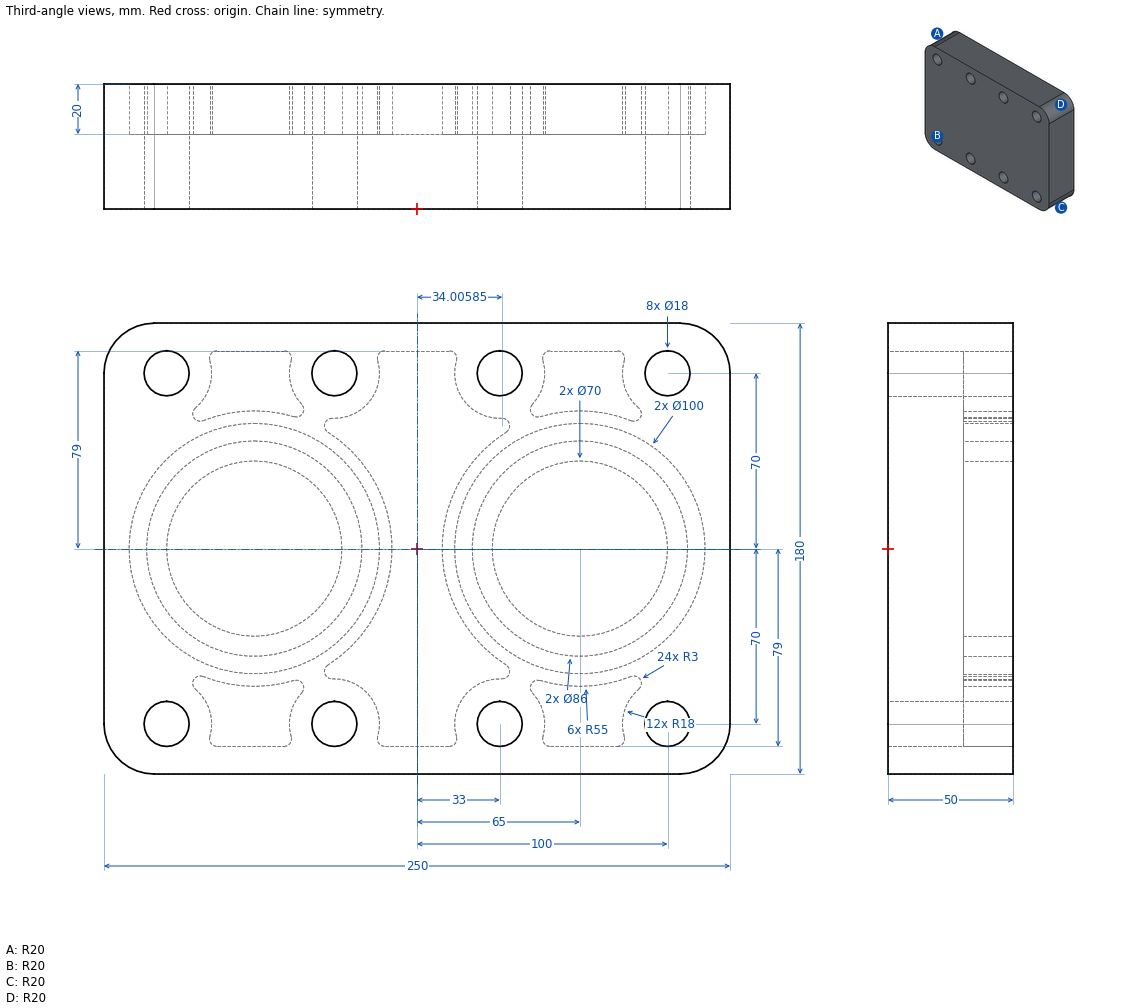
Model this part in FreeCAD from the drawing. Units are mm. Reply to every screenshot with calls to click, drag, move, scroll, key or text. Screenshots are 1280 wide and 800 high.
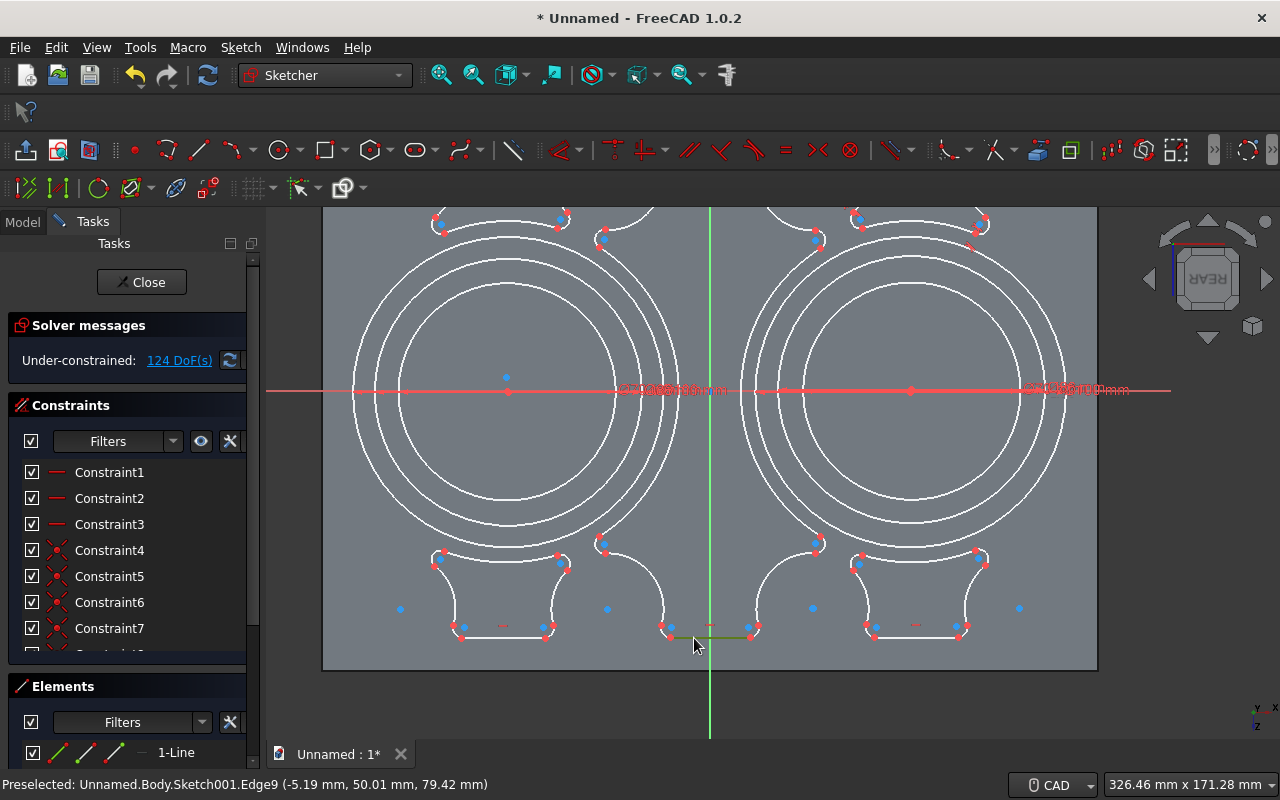
scroll(757, 633, up, 3)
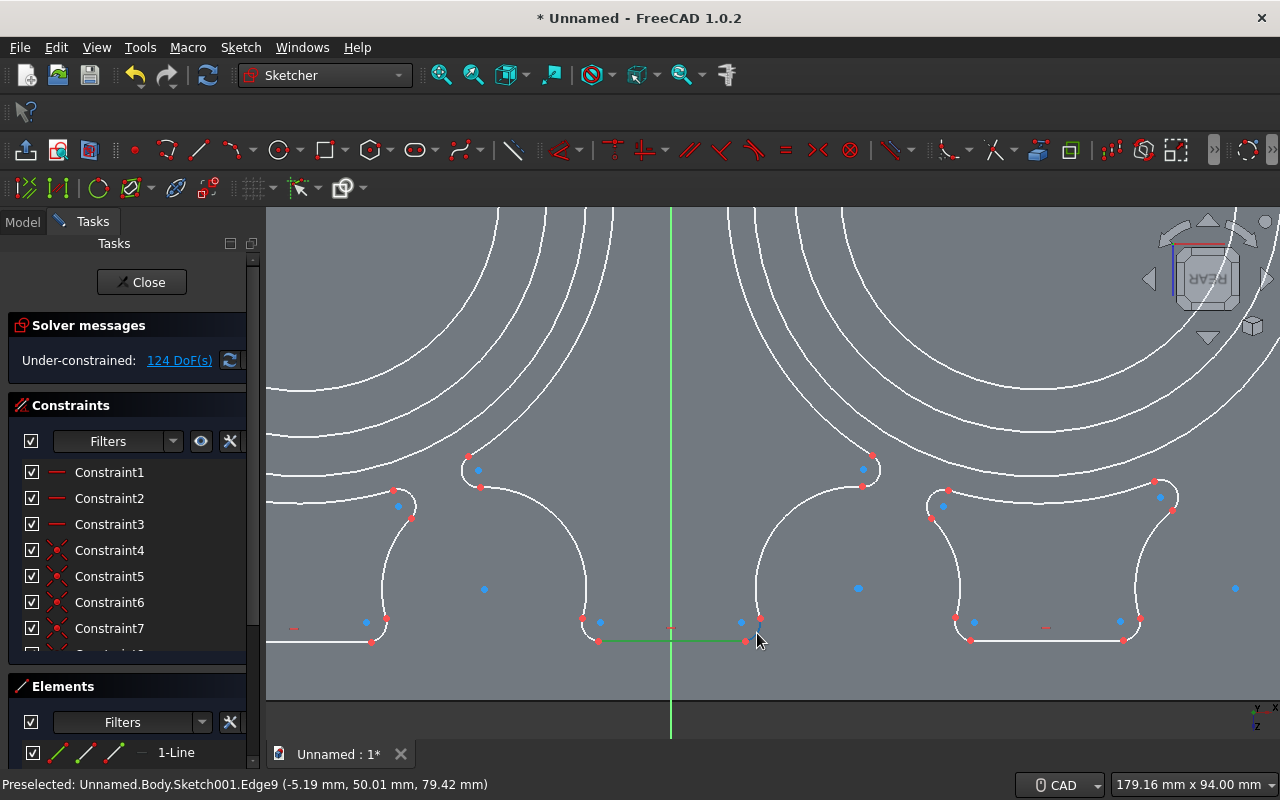
click(757, 633)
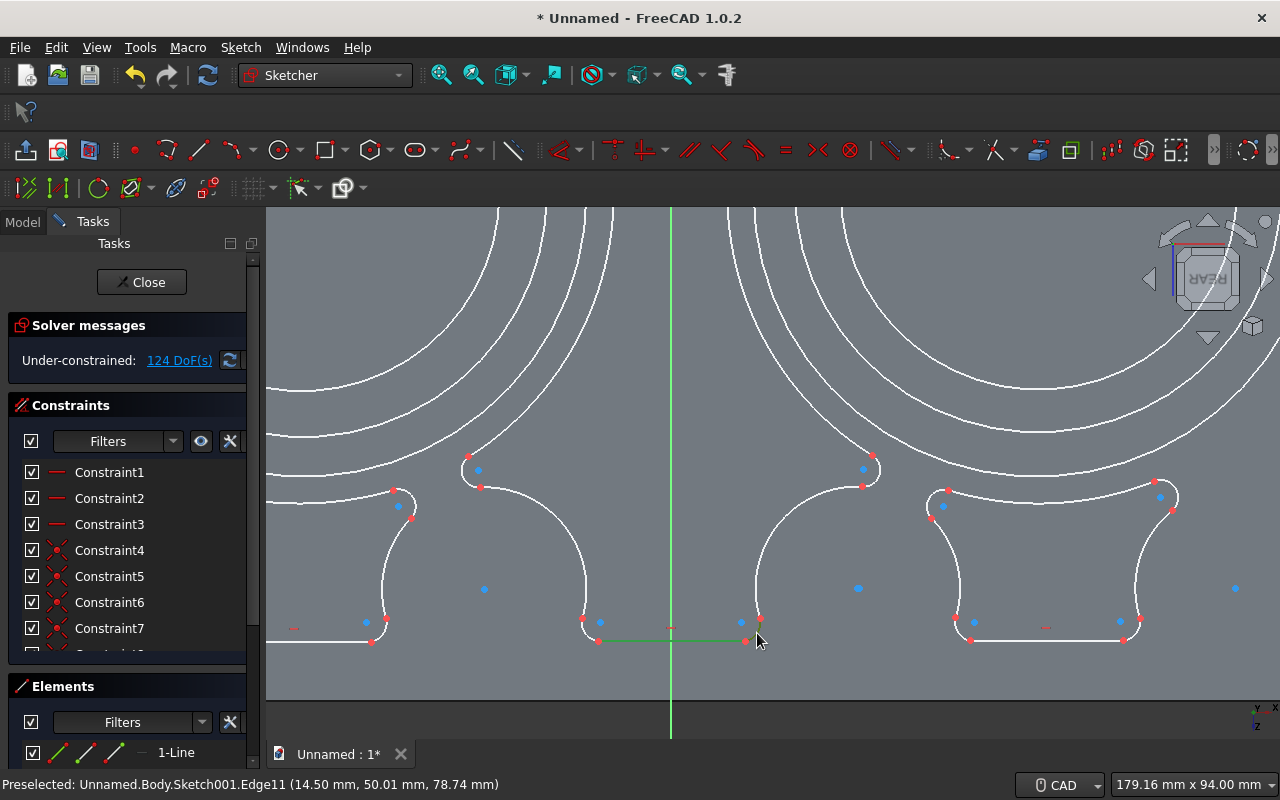
click(754, 150)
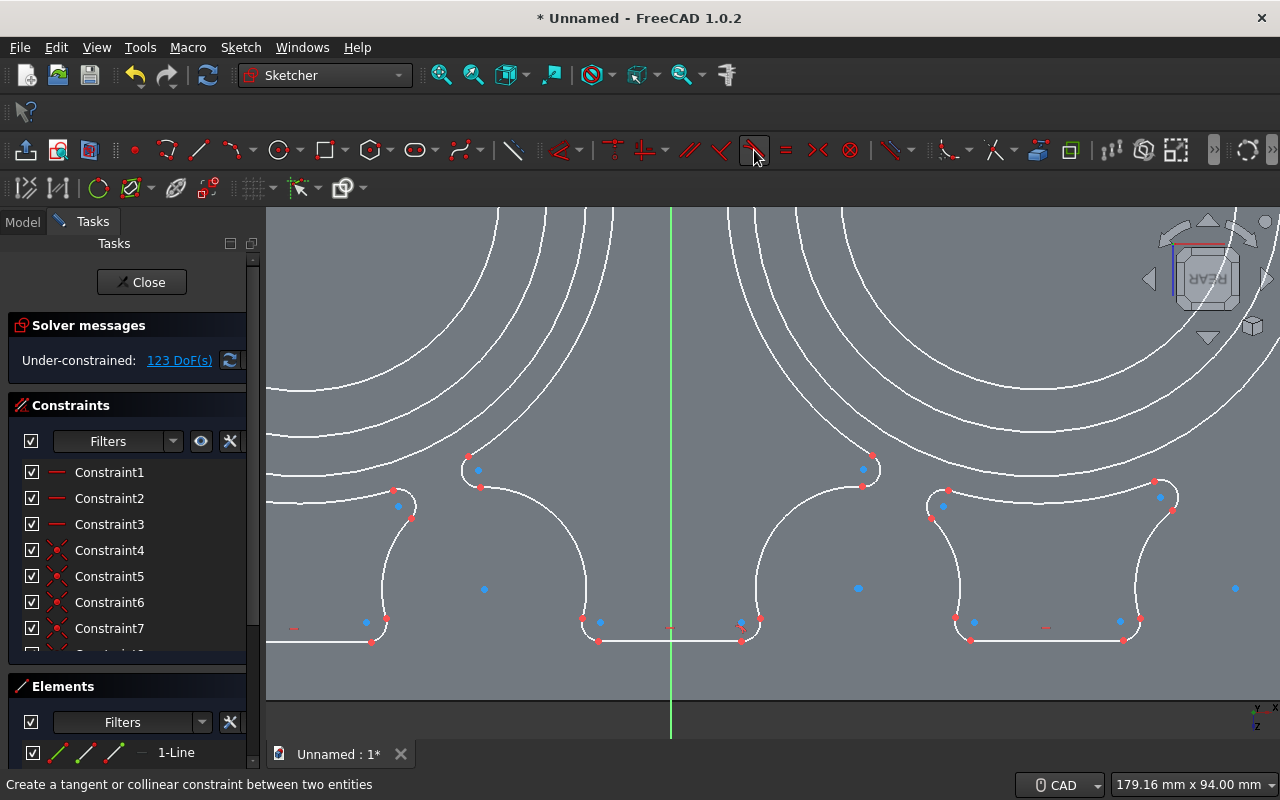
click(642, 641)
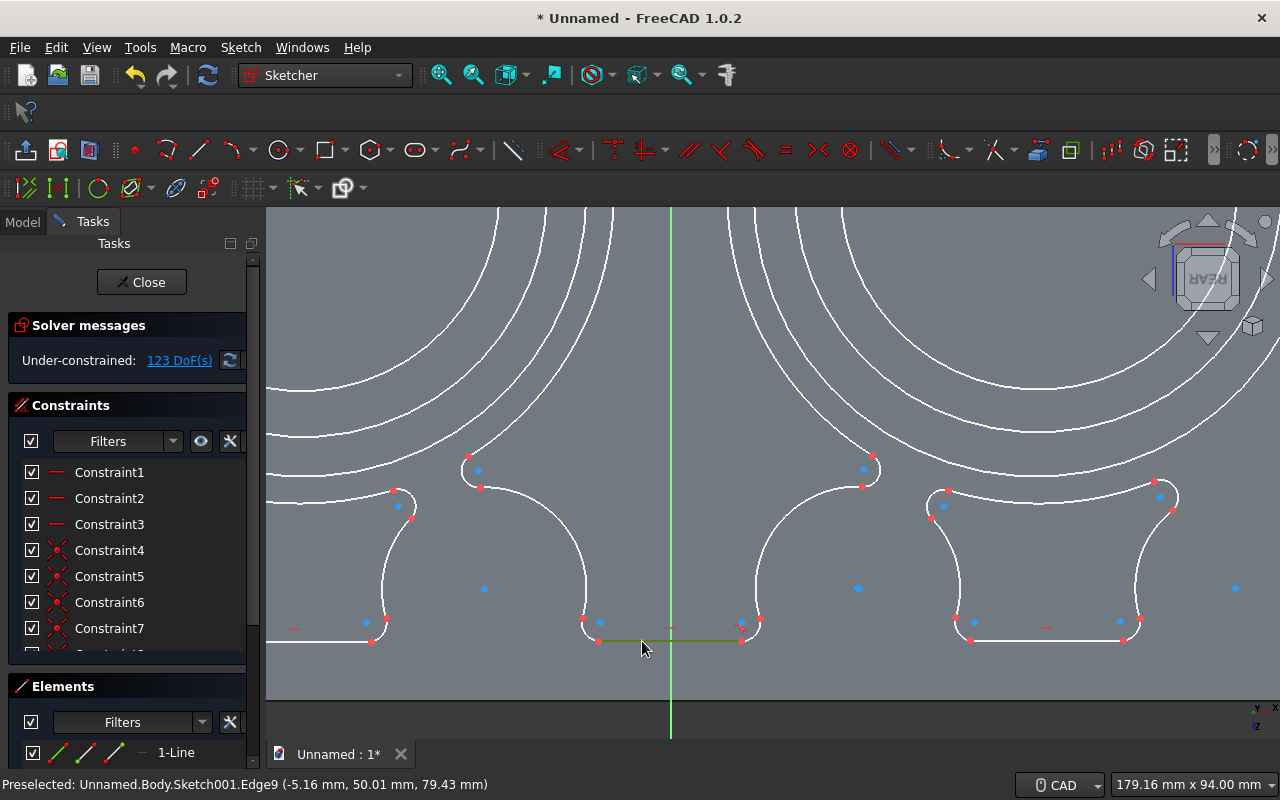
scroll(583, 628, up, 2)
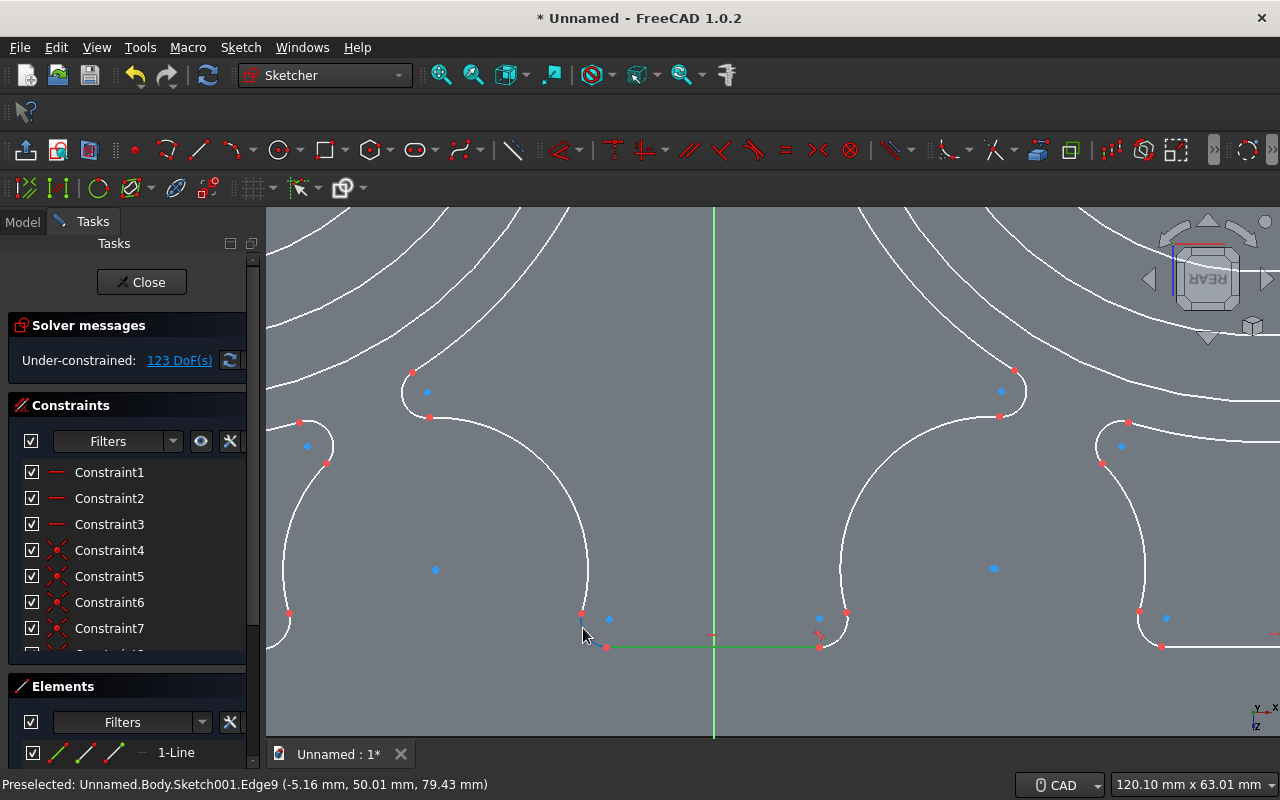
click(582, 627)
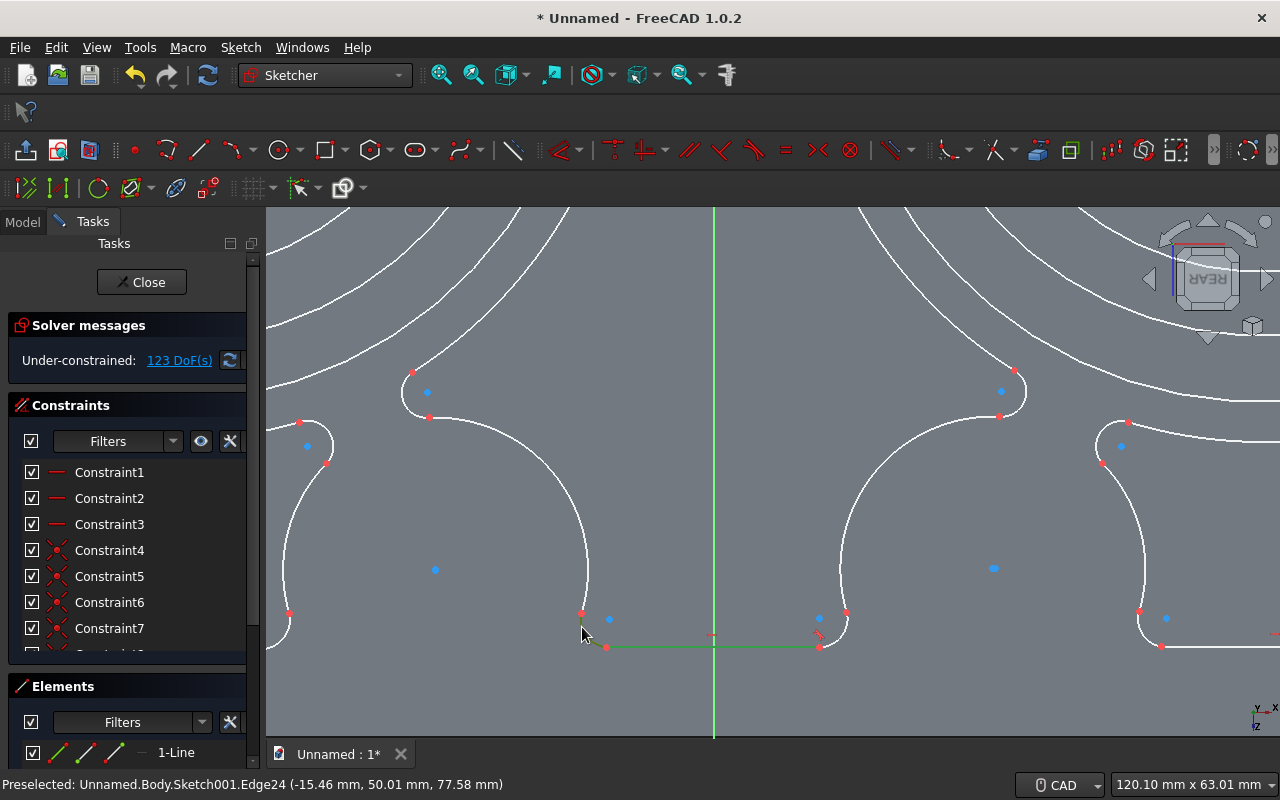
click(754, 150)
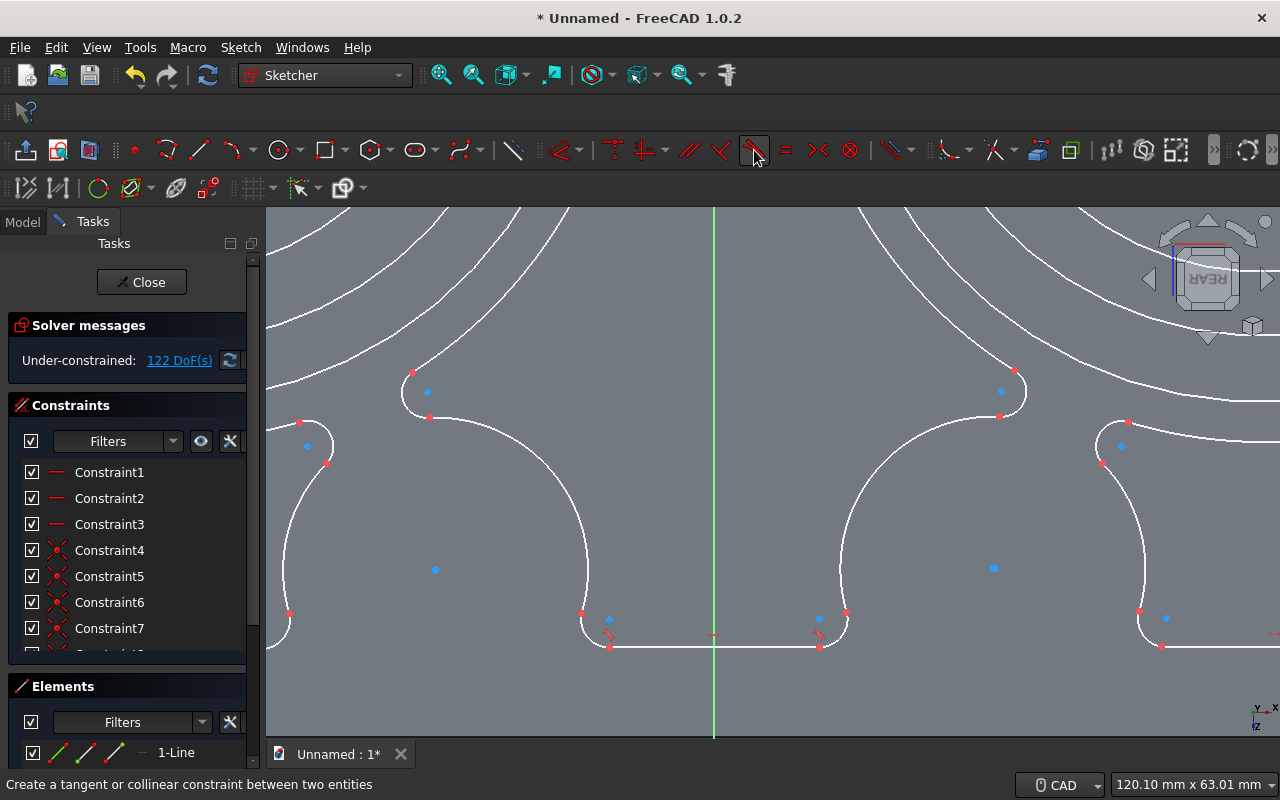
scroll(701, 635, down, 7)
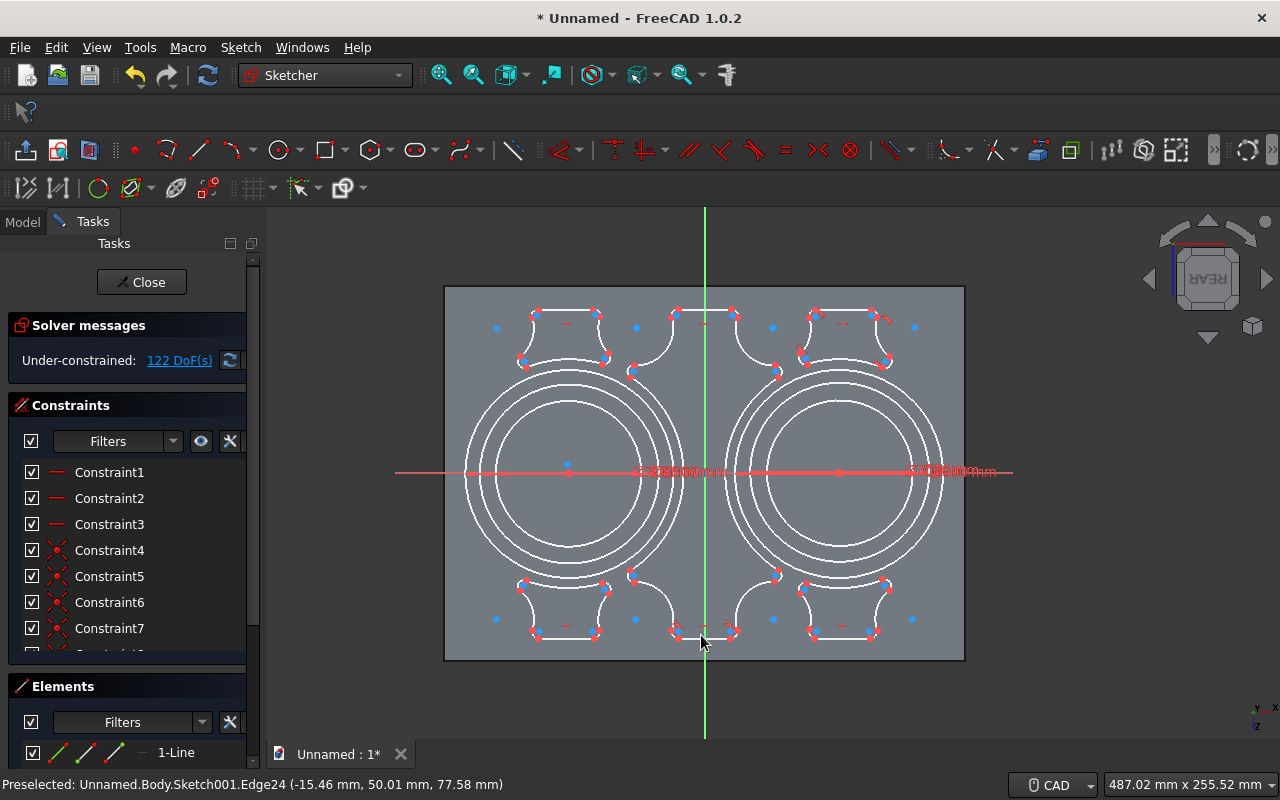
scroll(716, 310, up, 2)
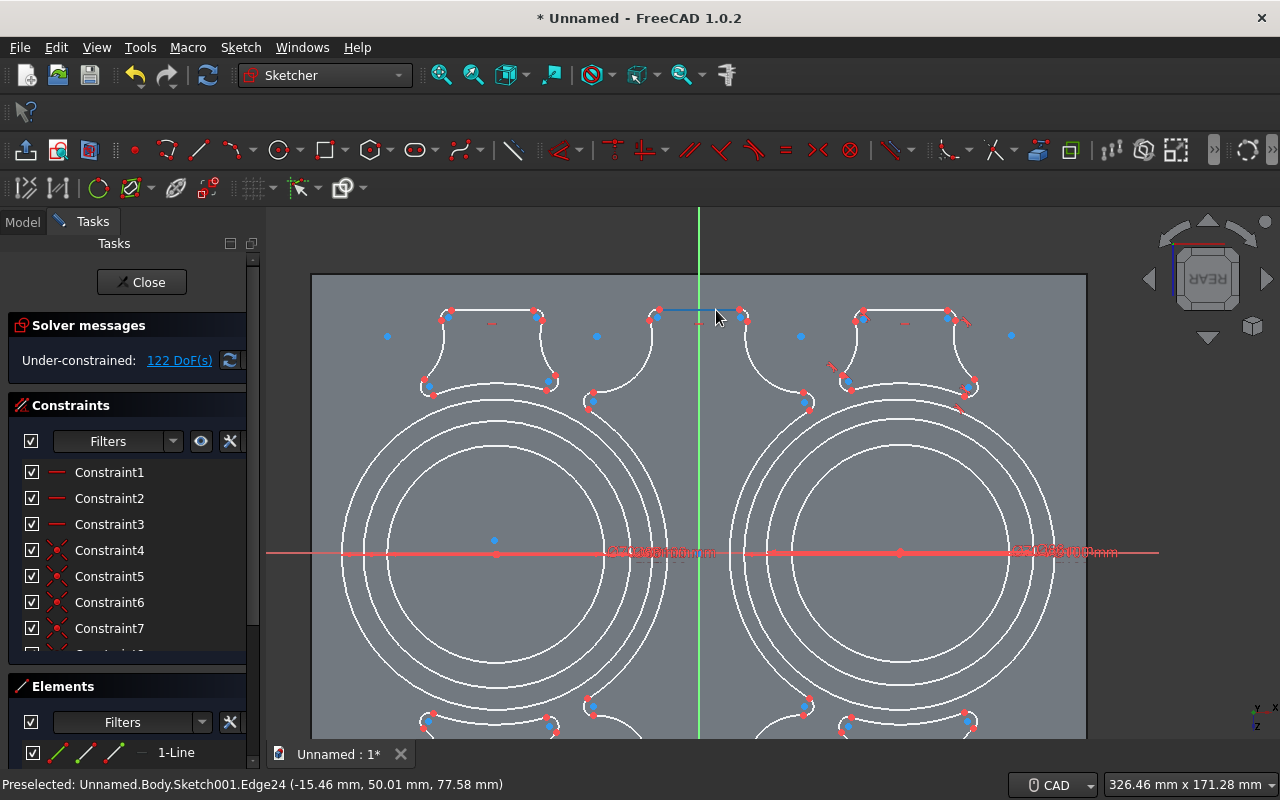
click(715, 310)